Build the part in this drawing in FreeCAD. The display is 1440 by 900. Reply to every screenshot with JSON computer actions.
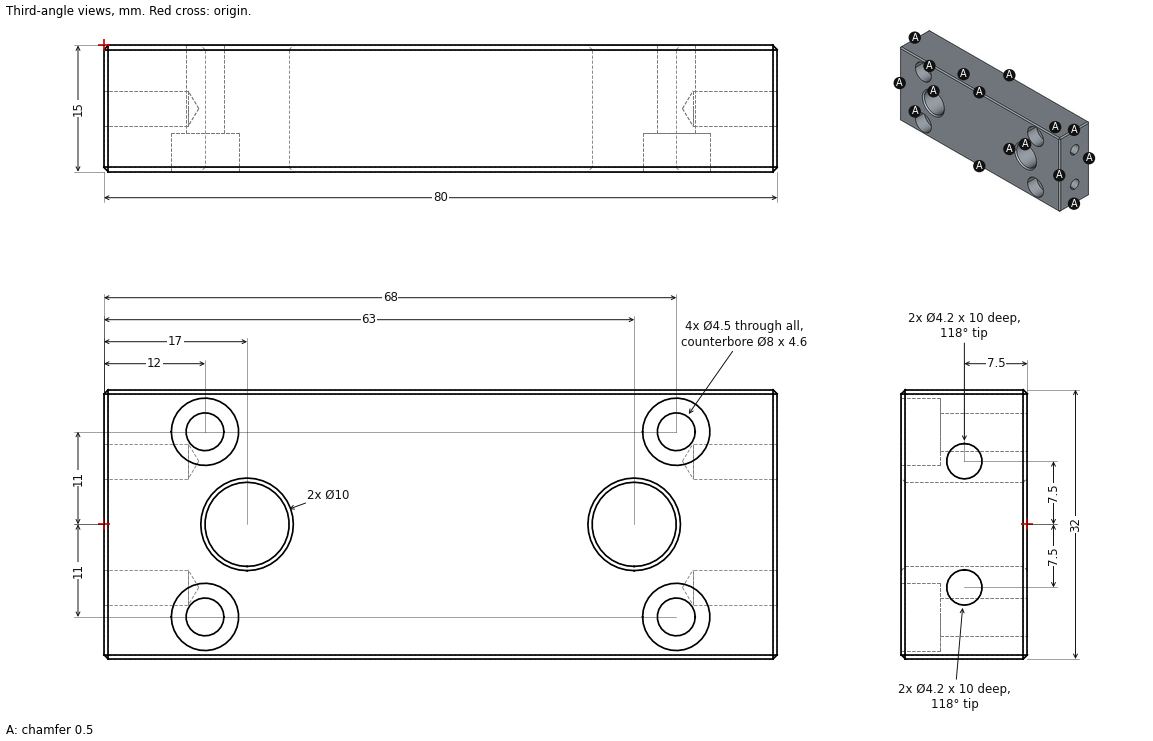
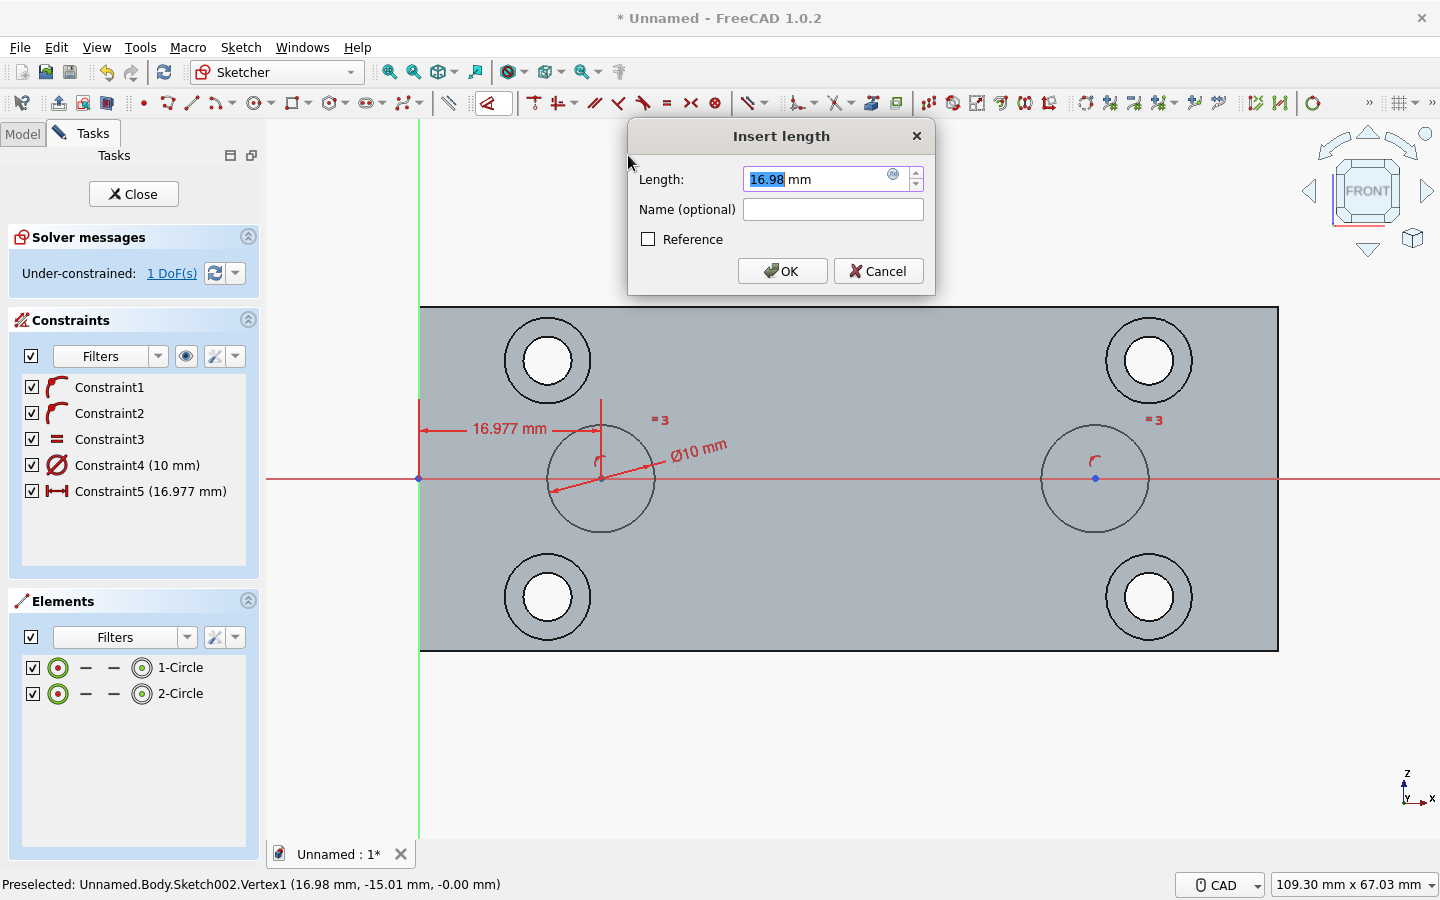
{"action": "type", "text": "17"}
{"action": "key", "text": "Return"}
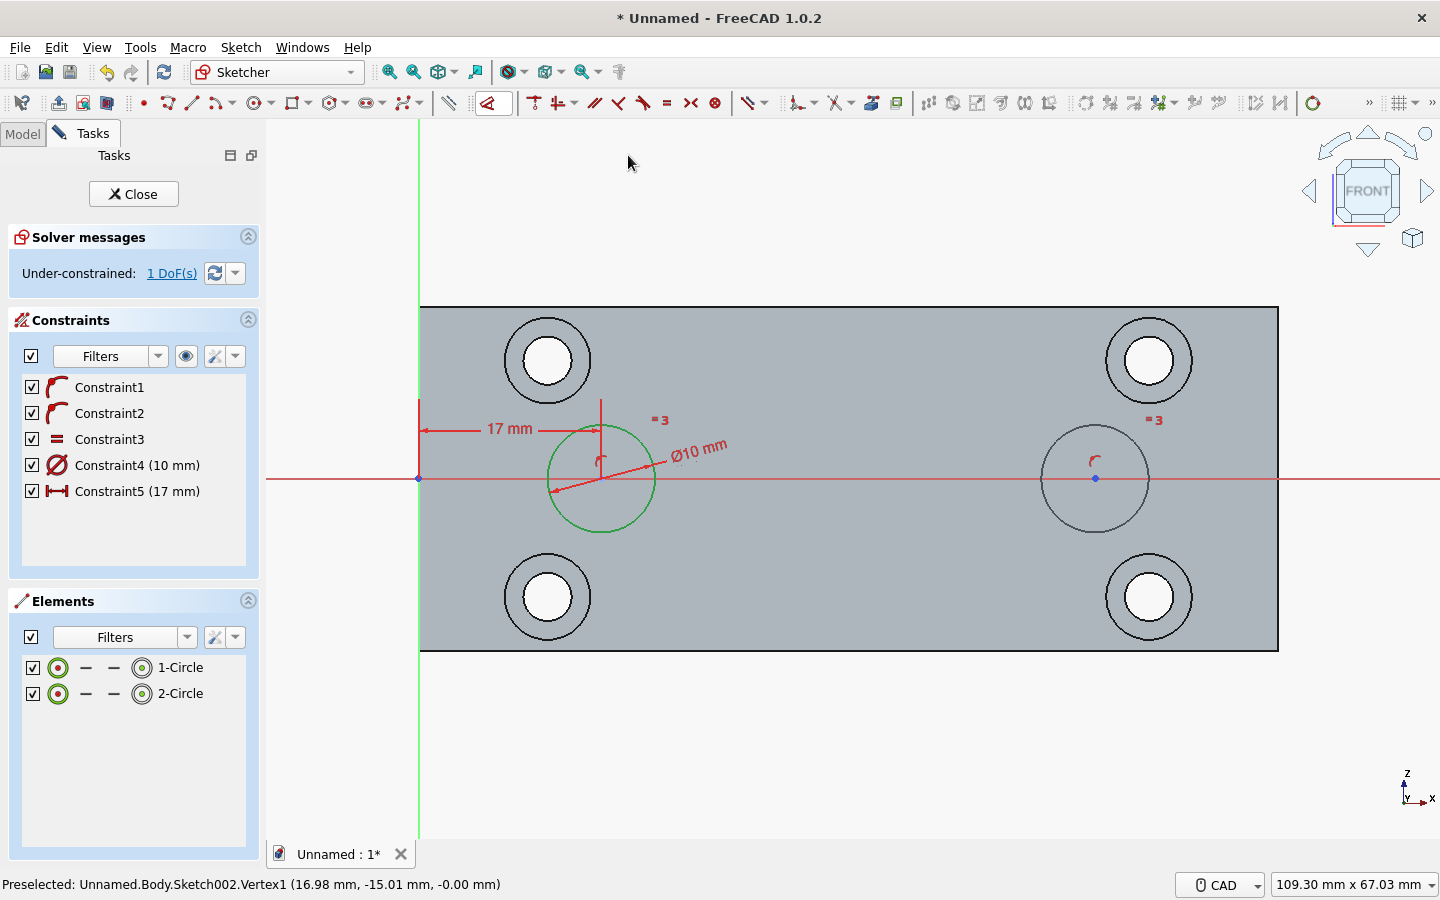
{"action": "left_click", "coordinate": [1095, 479]}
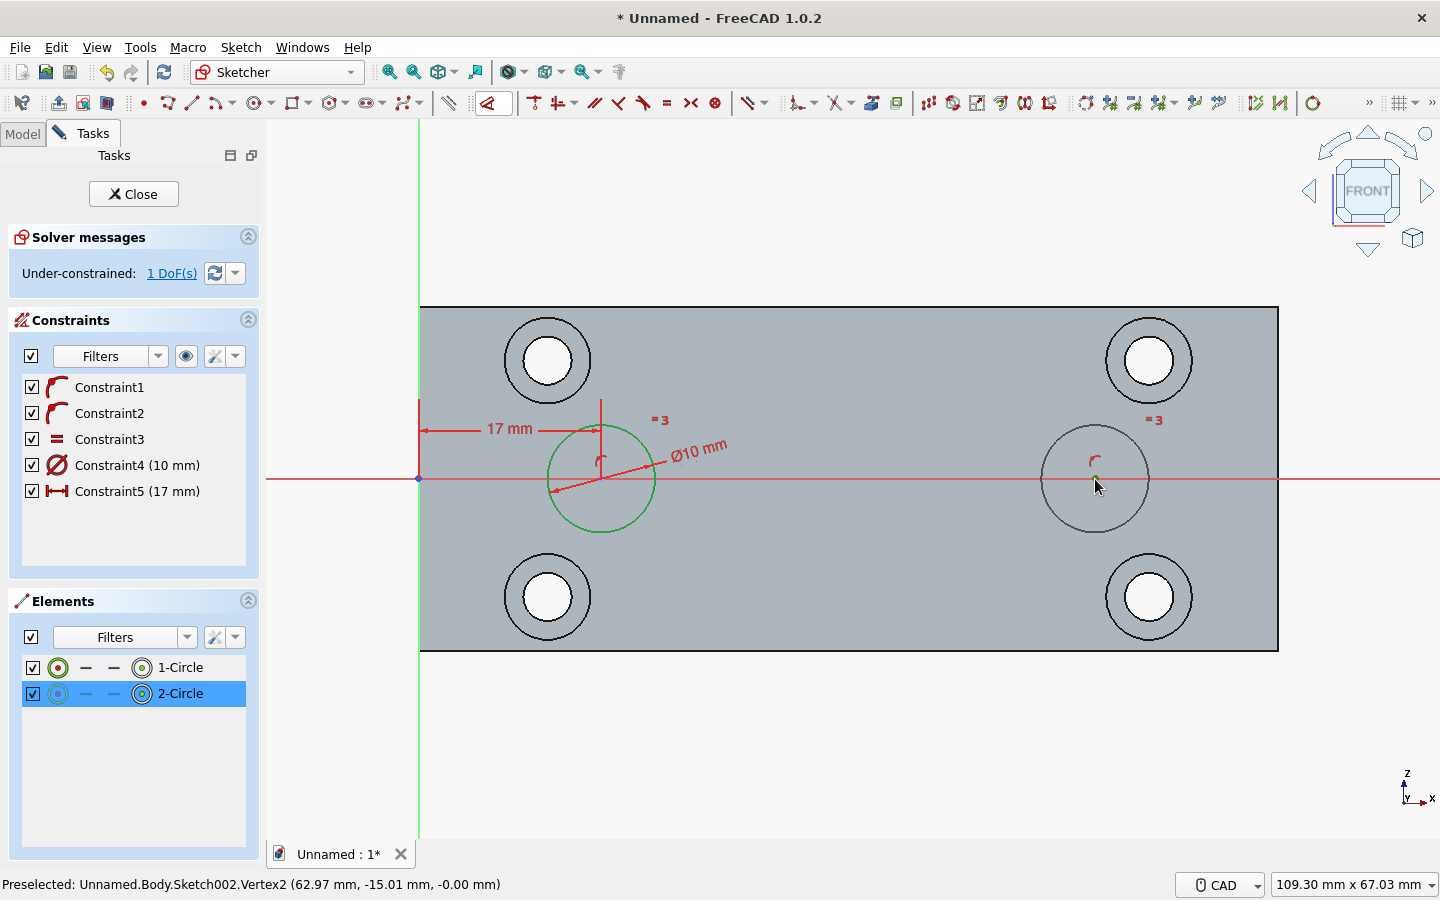
{"action": "left_click", "coordinate": [506, 104]}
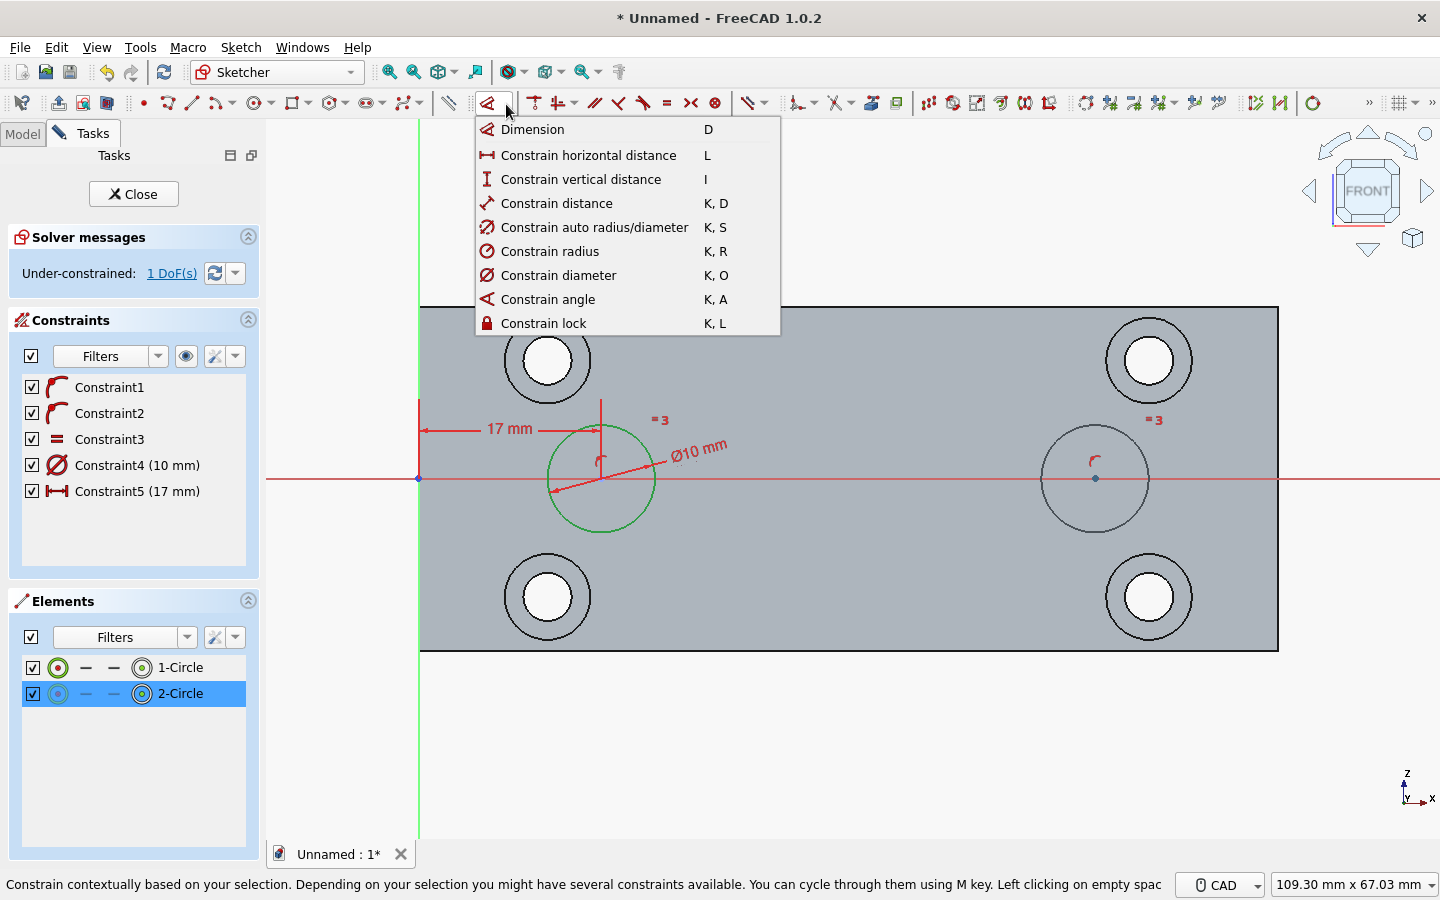
{"action": "left_click", "coordinate": [628, 155]}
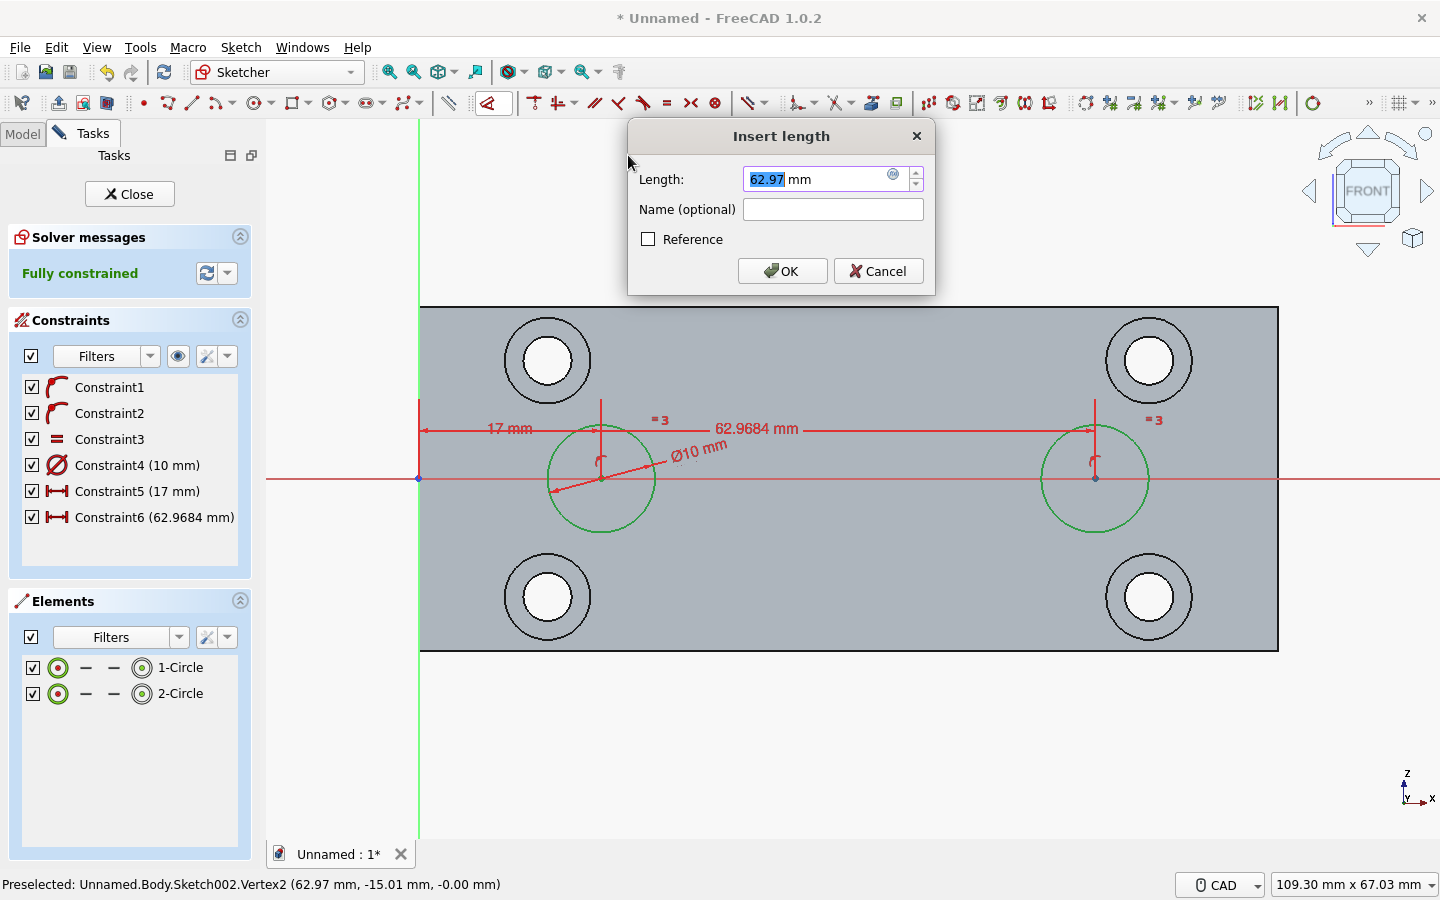
{"action": "type", "text": "63"}
{"action": "key", "text": "Return"}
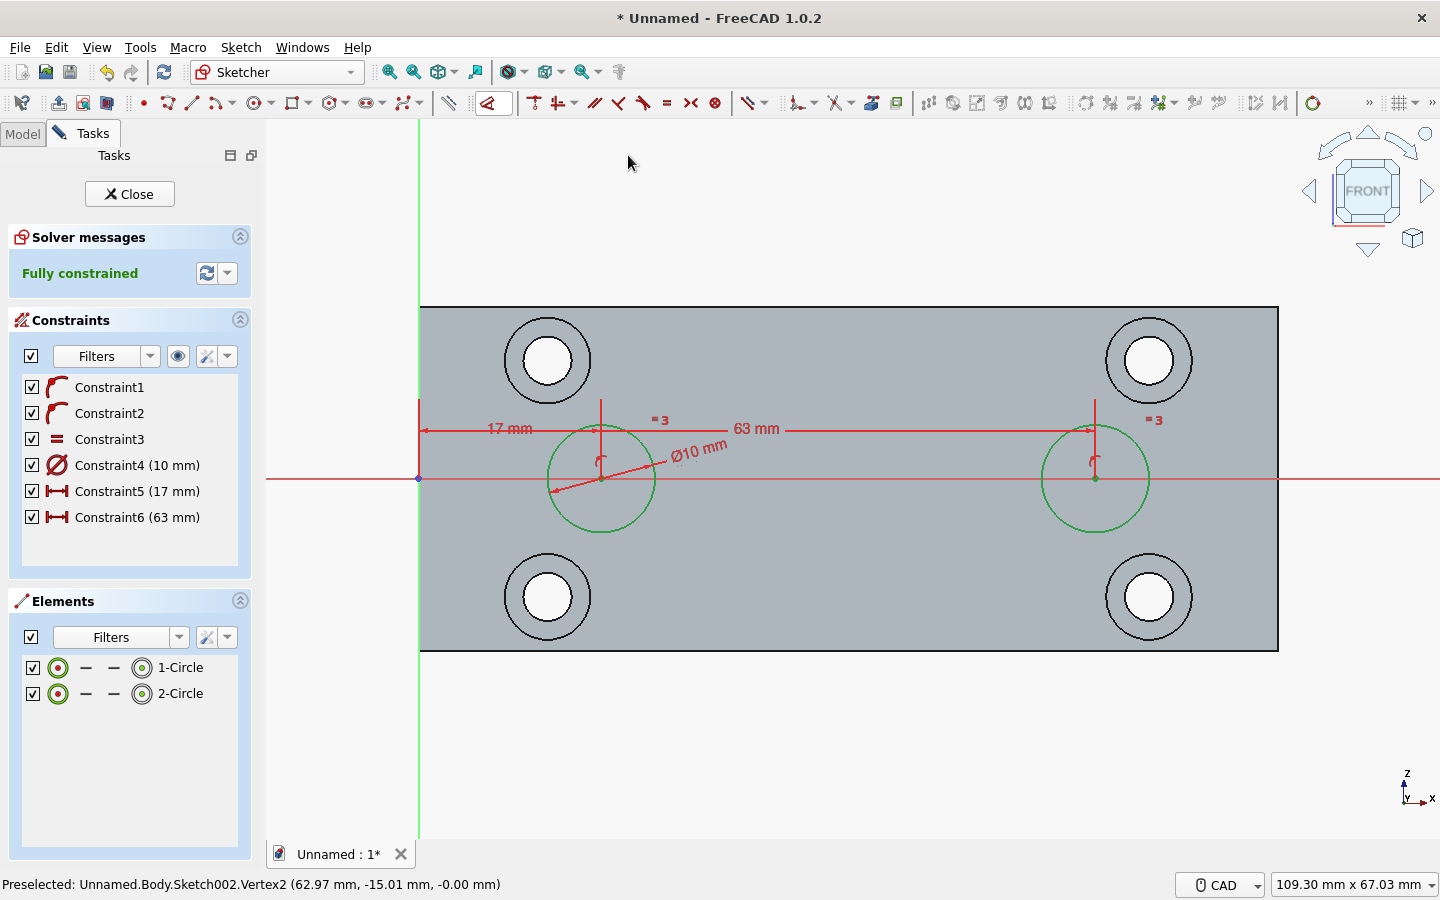
{"action": "left_click", "coordinate": [130, 194]}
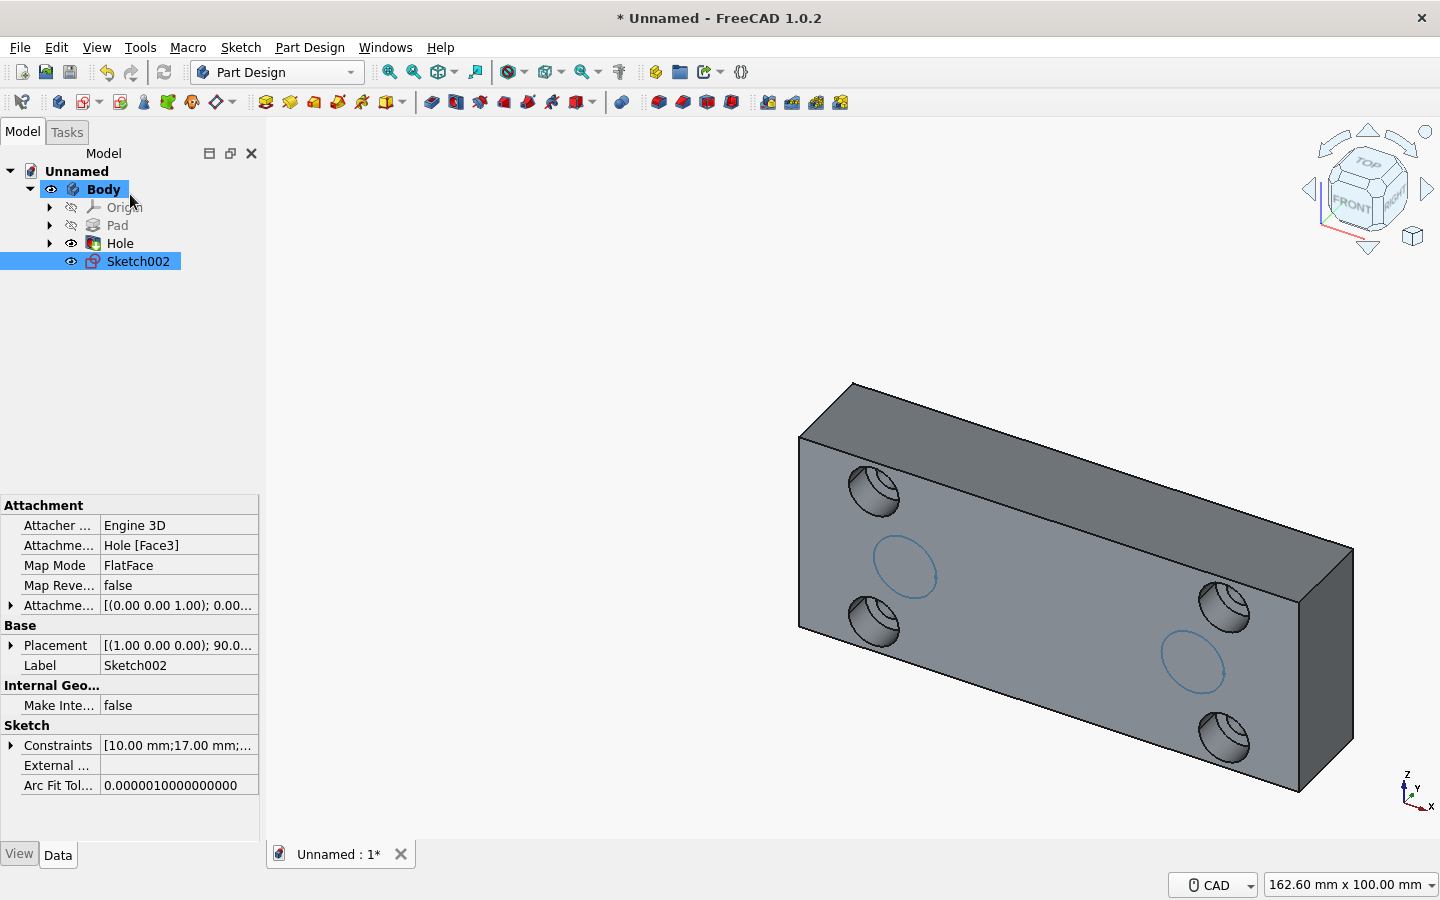
{"action": "left_click", "coordinate": [432, 102]}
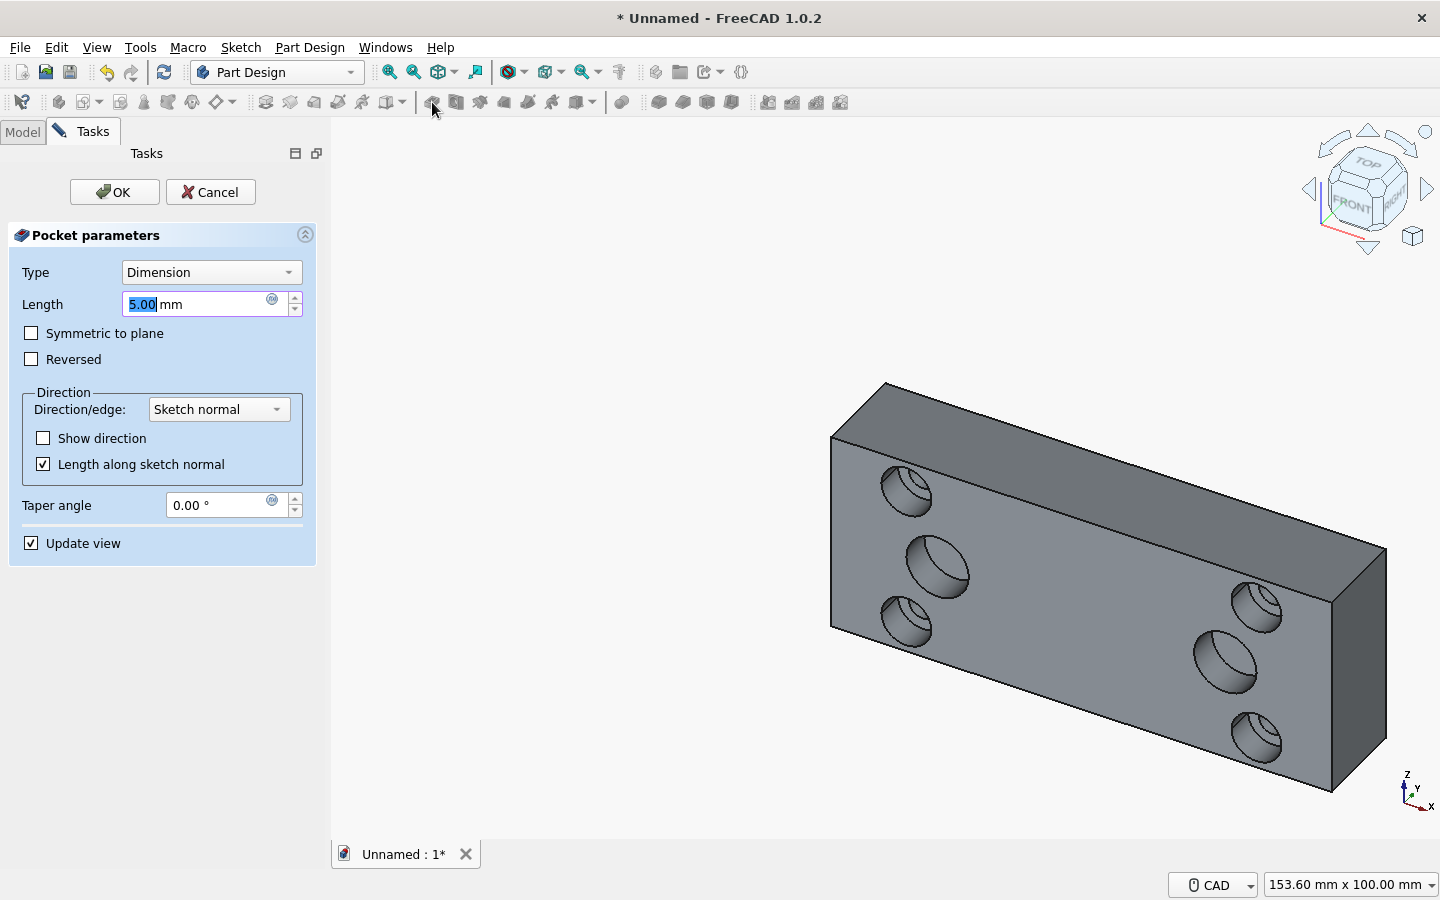
{"action": "left_click", "coordinate": [212, 272]}